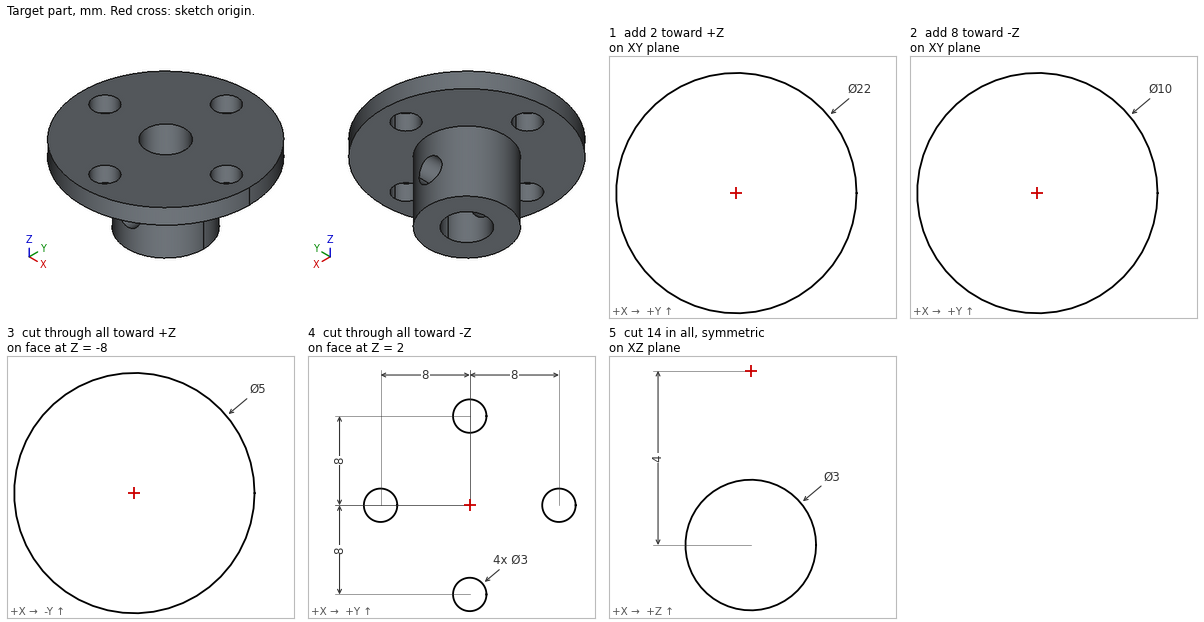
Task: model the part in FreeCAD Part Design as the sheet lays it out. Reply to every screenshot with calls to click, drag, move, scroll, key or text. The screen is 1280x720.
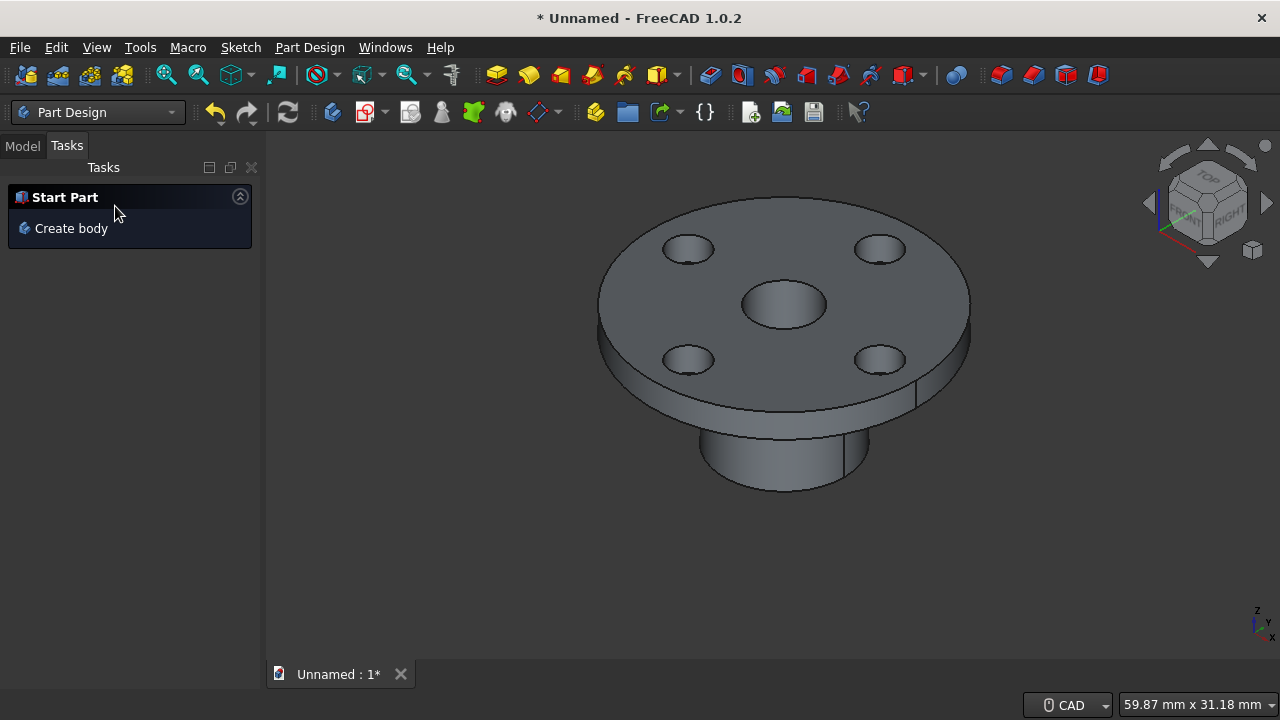
click(366, 112)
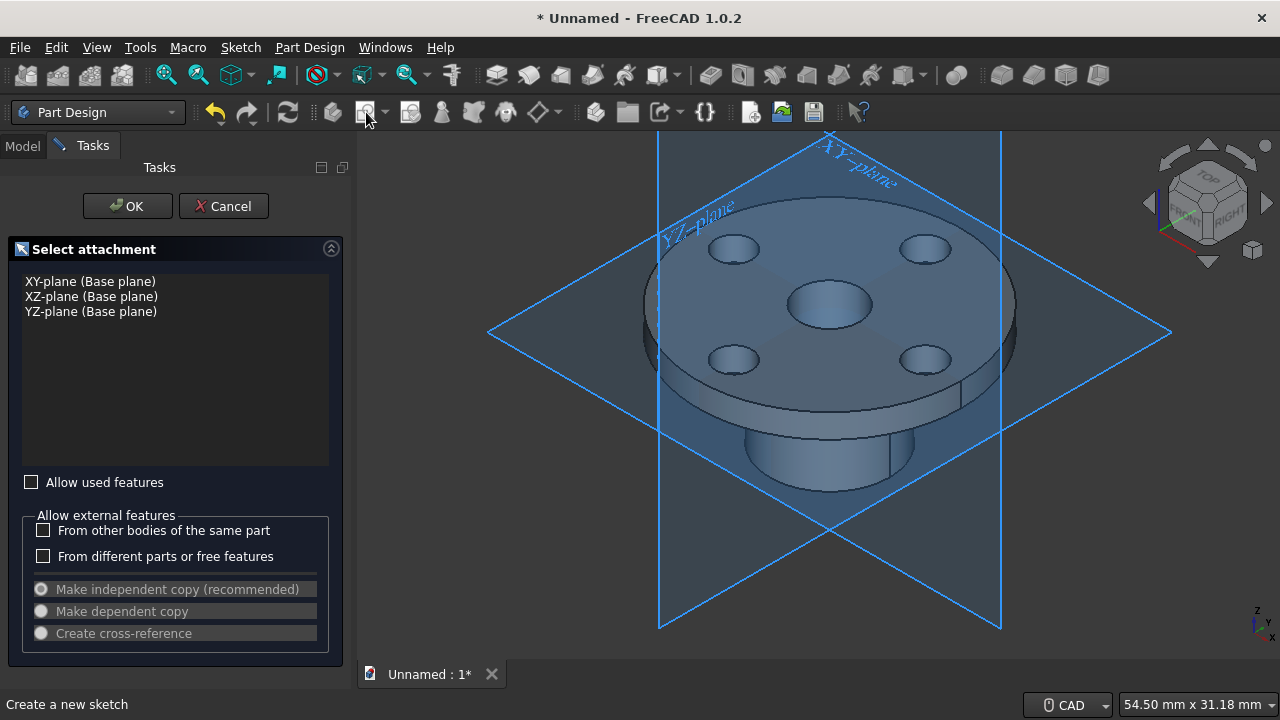
click(82, 296)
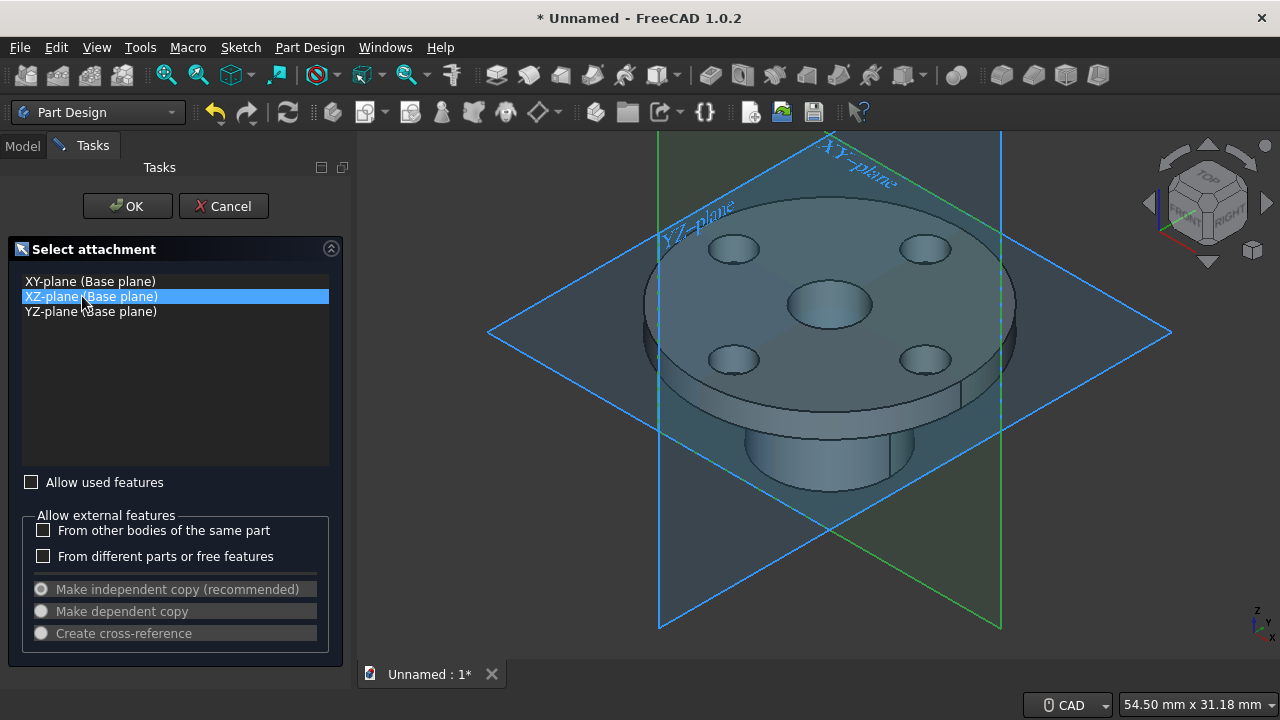
click(128, 206)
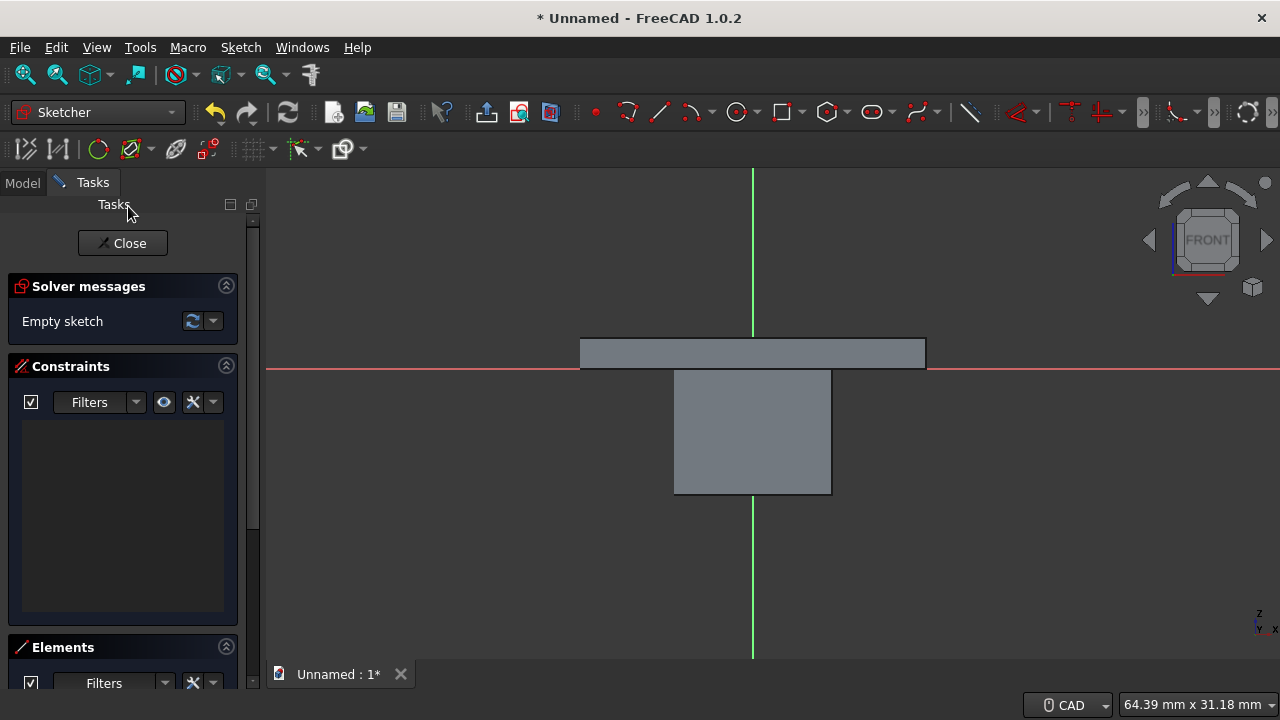
click(552, 112)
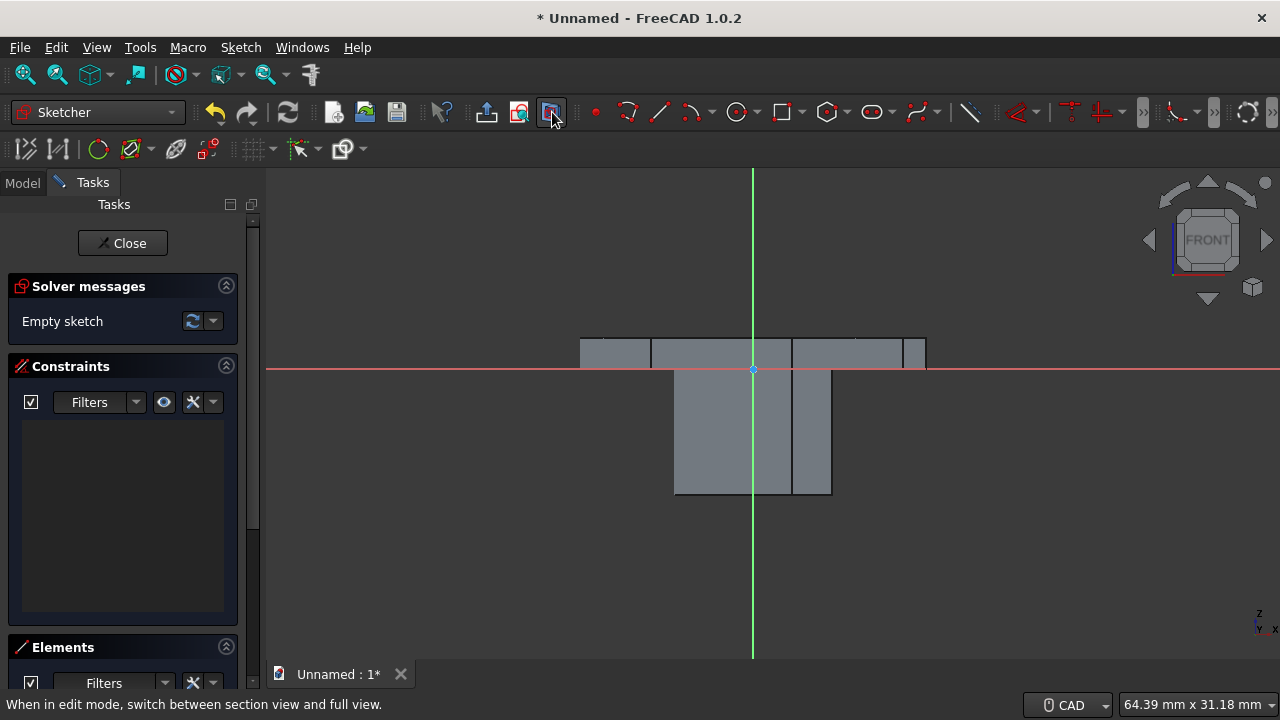
scroll(774, 412, up, 6)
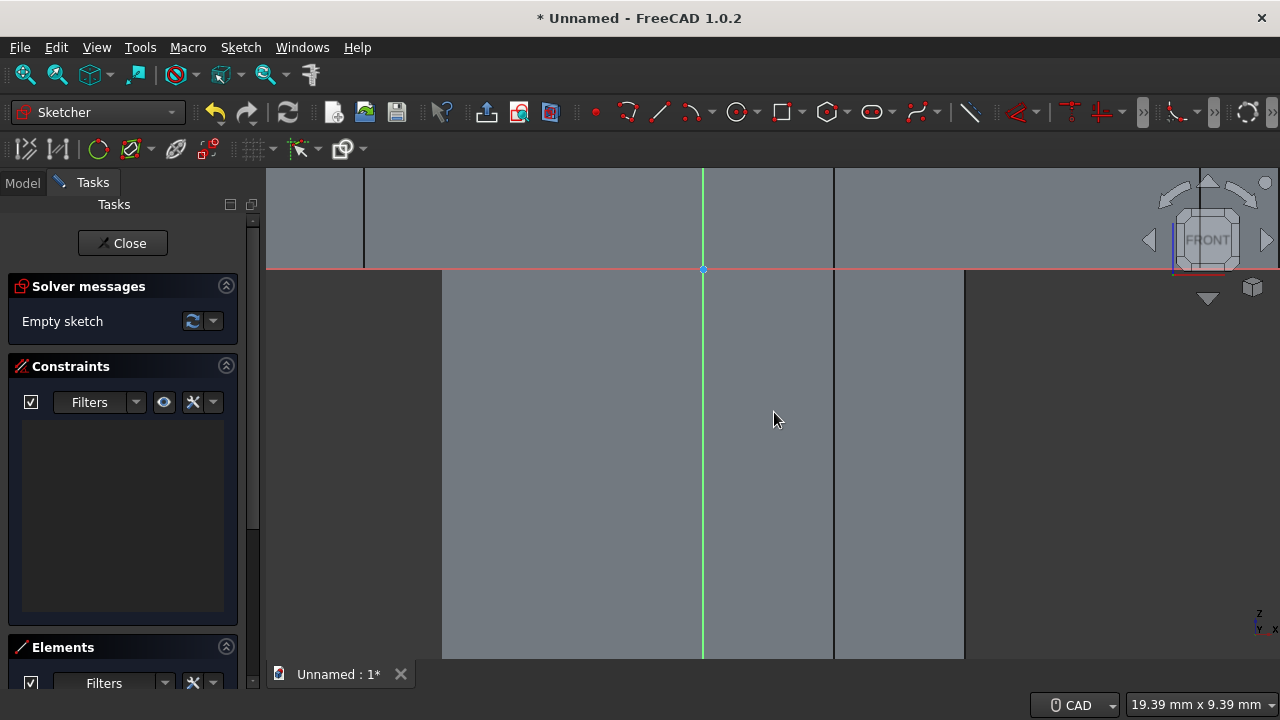
key(g)
key(c)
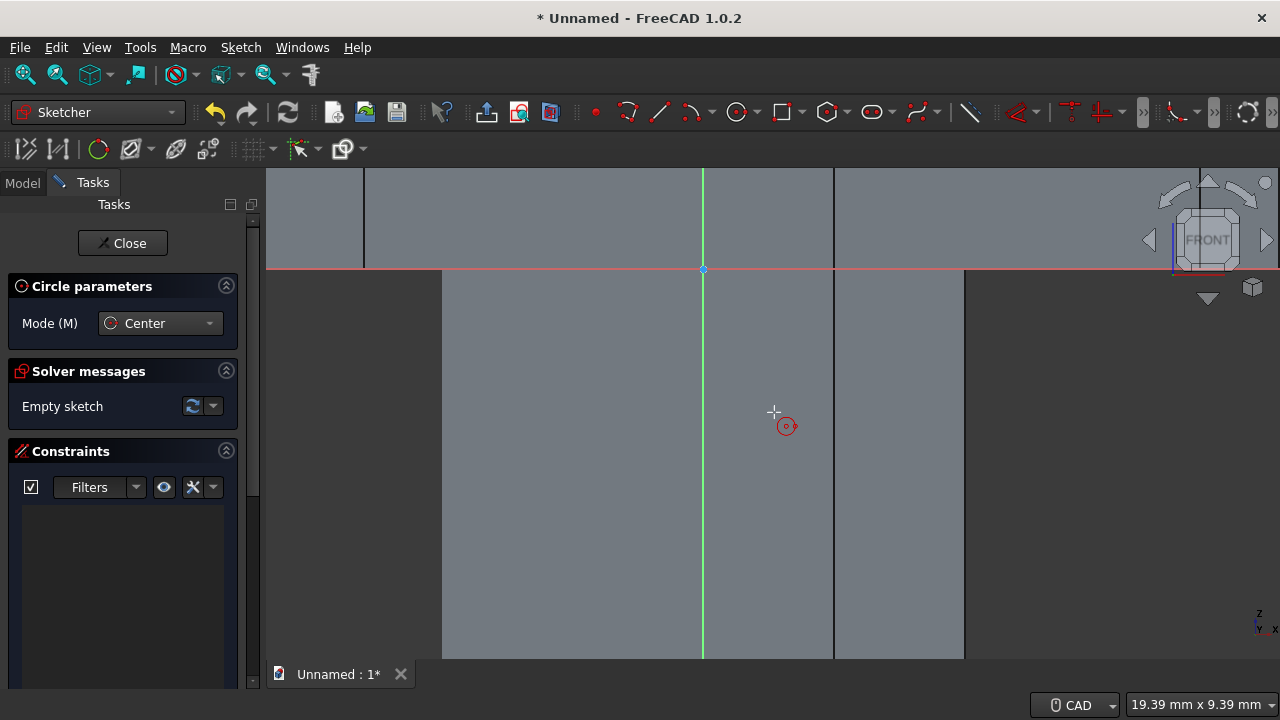
click(703, 478)
click(759, 423)
key(Escape)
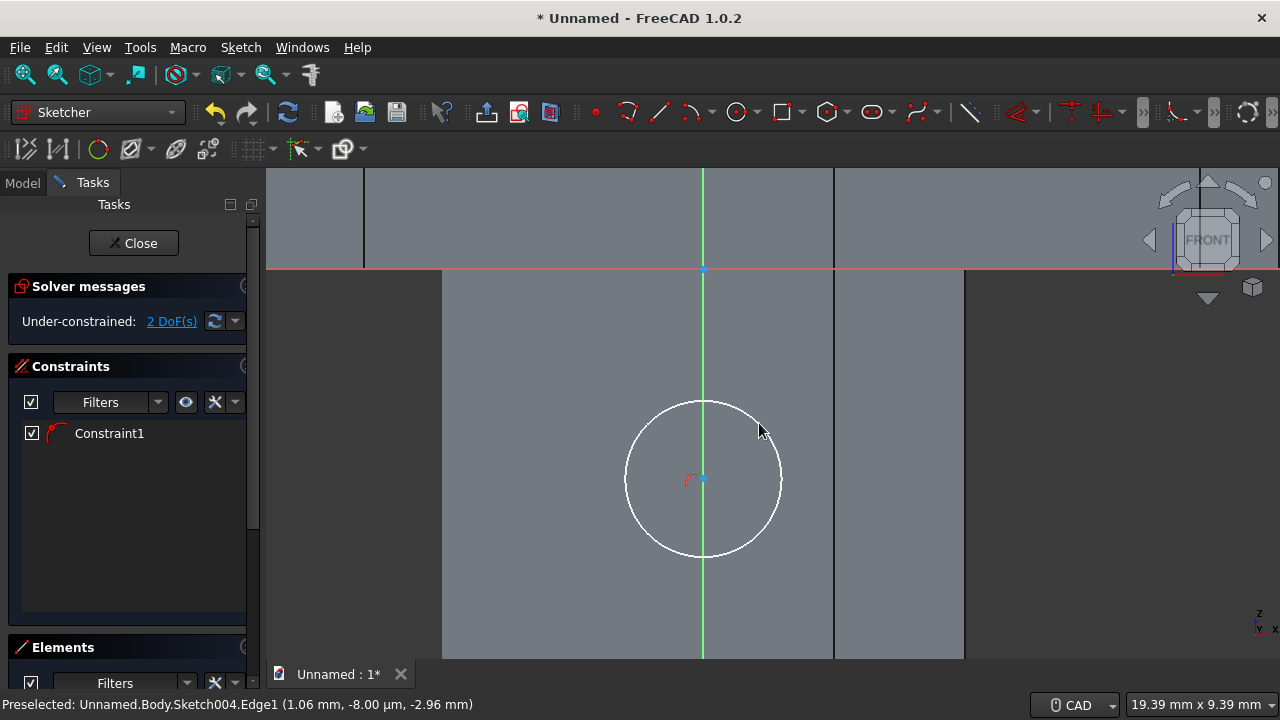
click(759, 424)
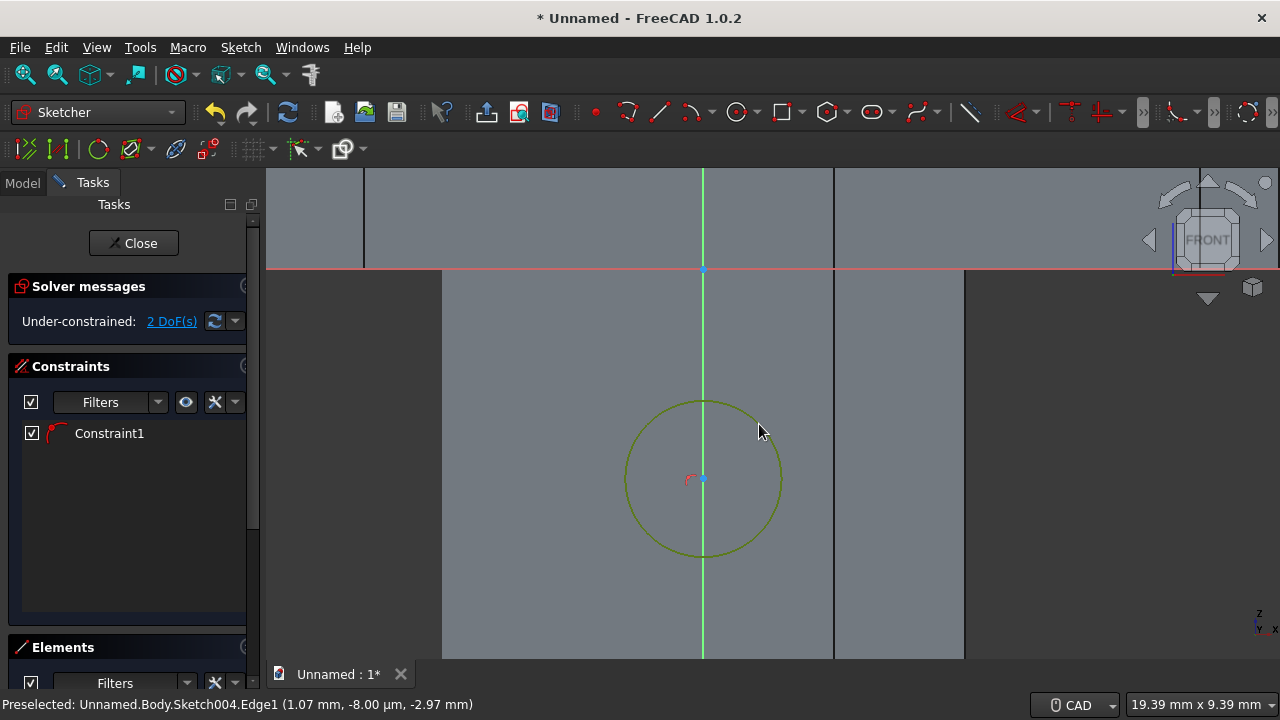
key(k)
key(o)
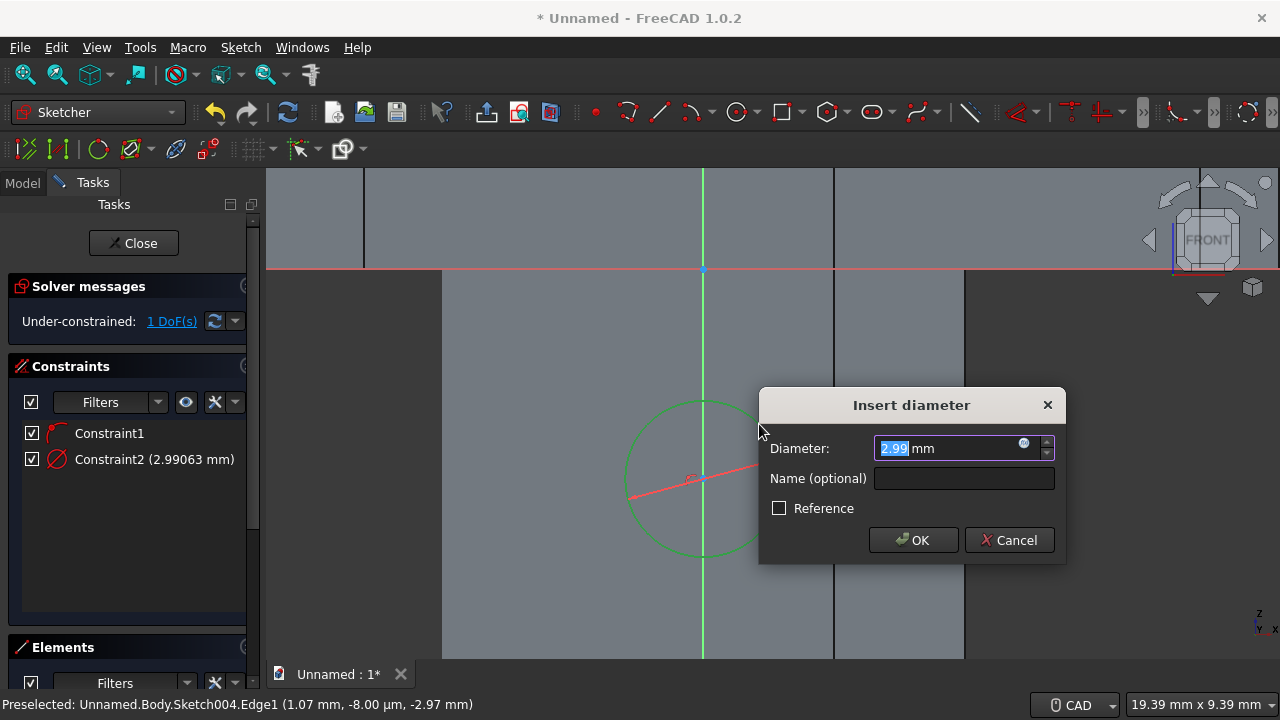
text(3)
key(Return)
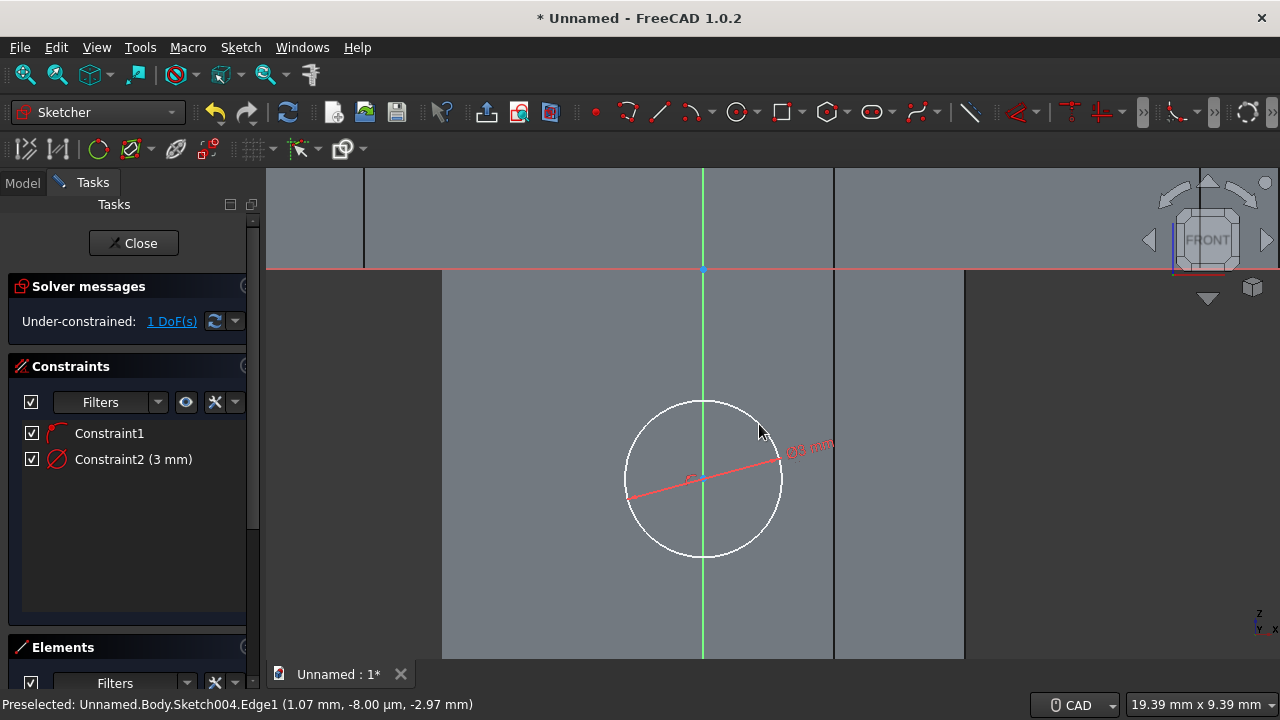
click(703, 479)